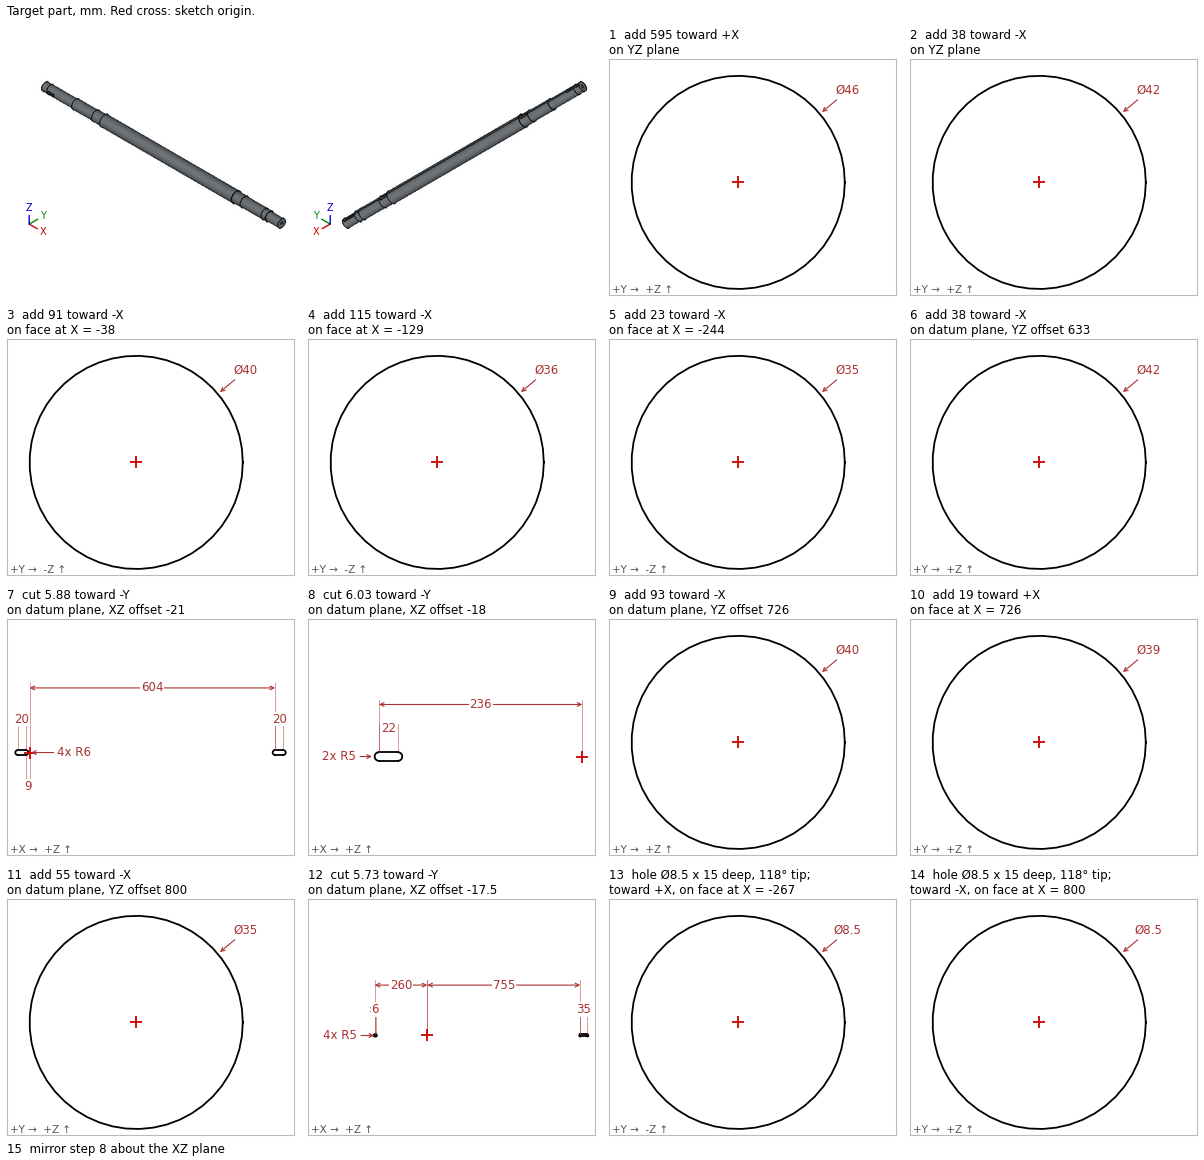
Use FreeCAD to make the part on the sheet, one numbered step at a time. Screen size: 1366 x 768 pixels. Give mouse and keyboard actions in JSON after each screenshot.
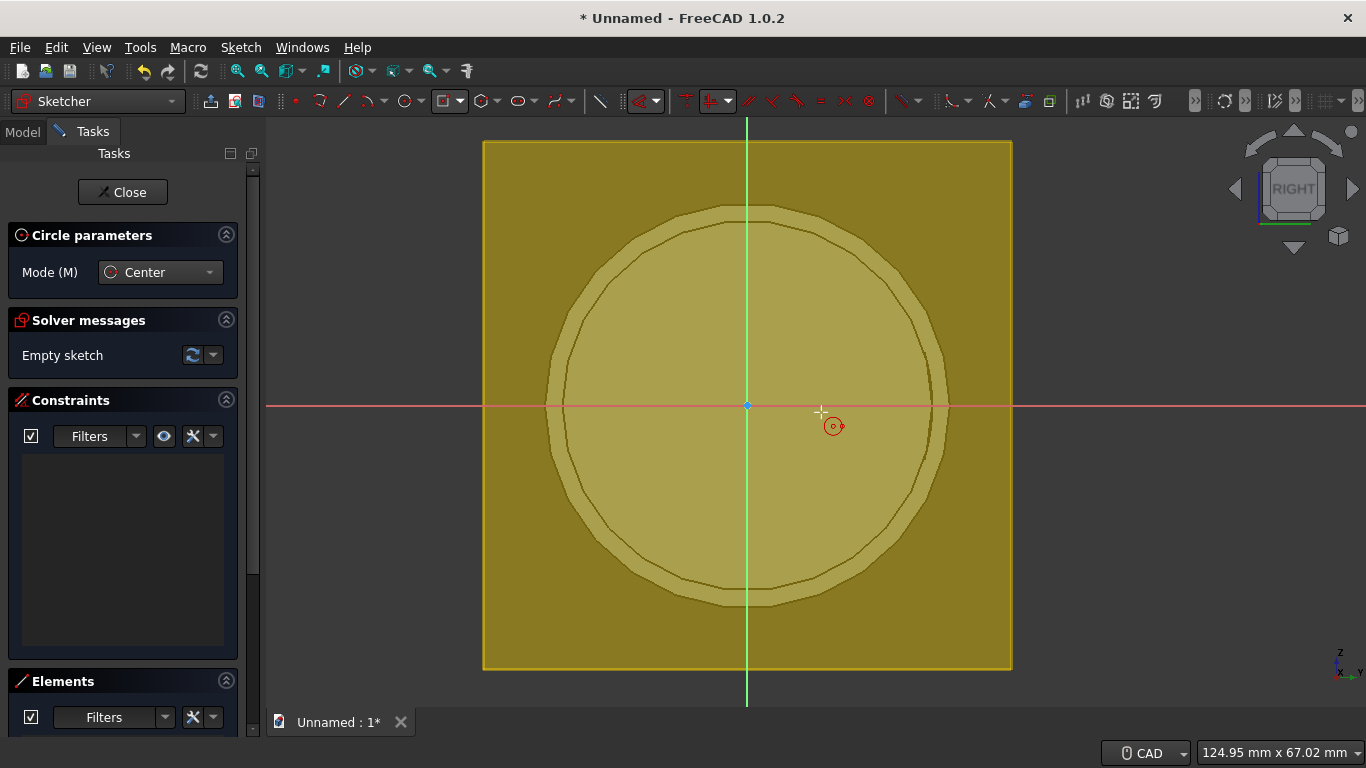
{"action": "left_click", "coordinate": [747, 406]}
{"action": "mouse_move", "coordinate": [872, 281]}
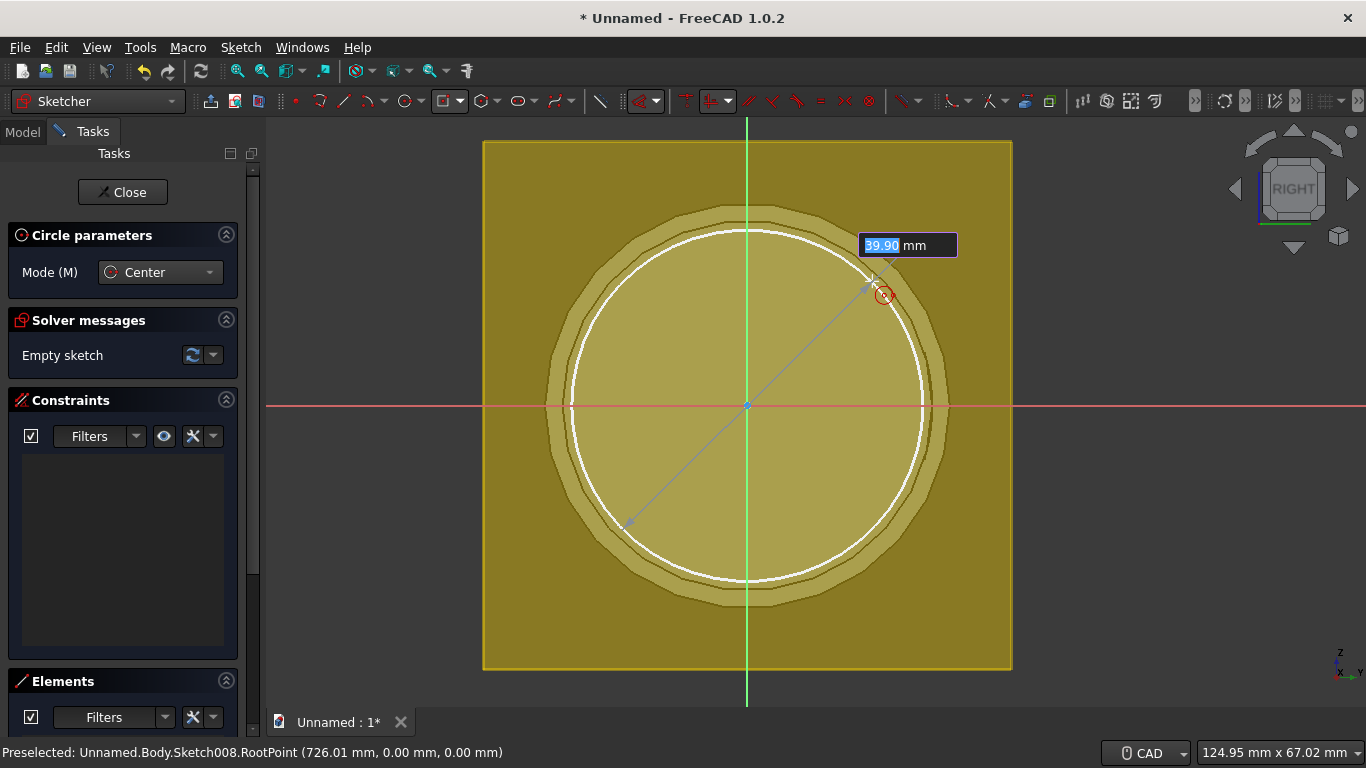
{"action": "type", "text": "40"}
{"action": "key", "text": "Return"}
{"action": "key", "text": "Escape"}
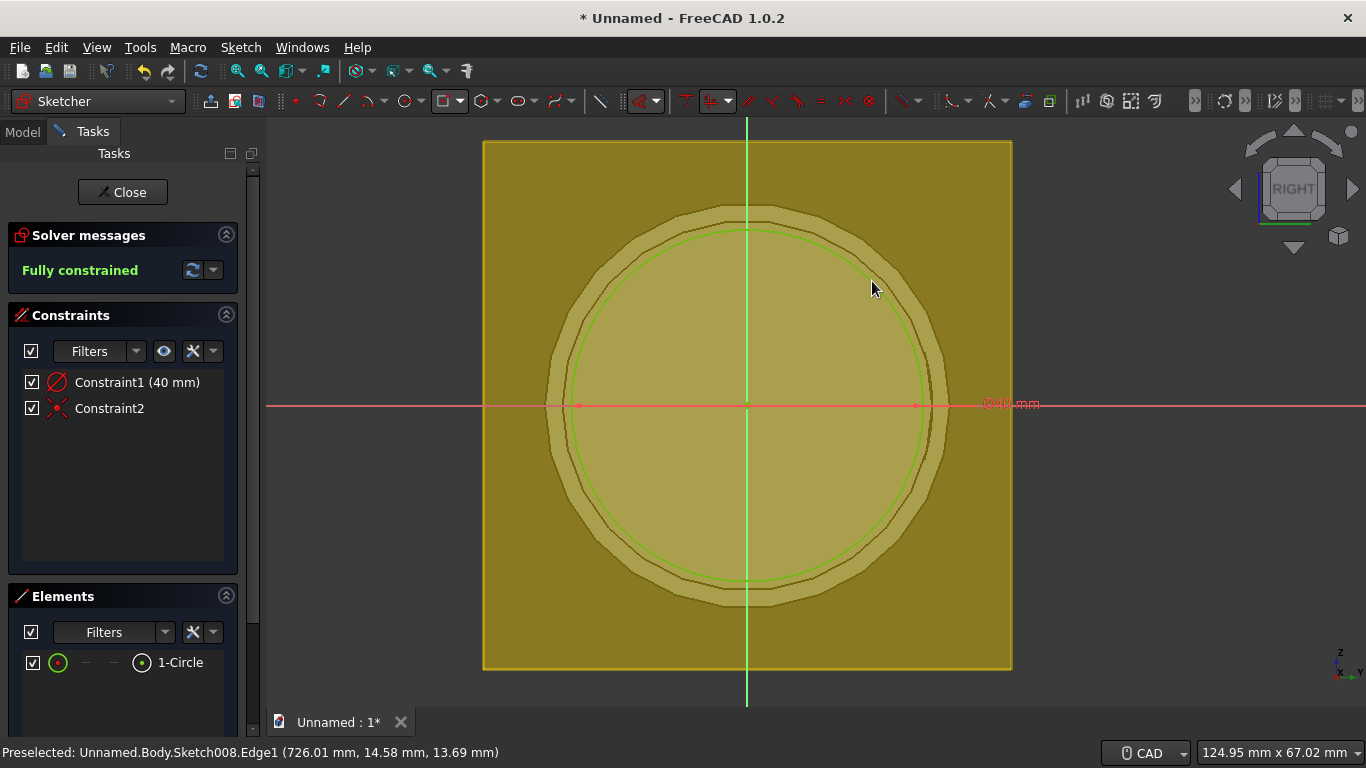
{"action": "left_click", "coordinate": [123, 192]}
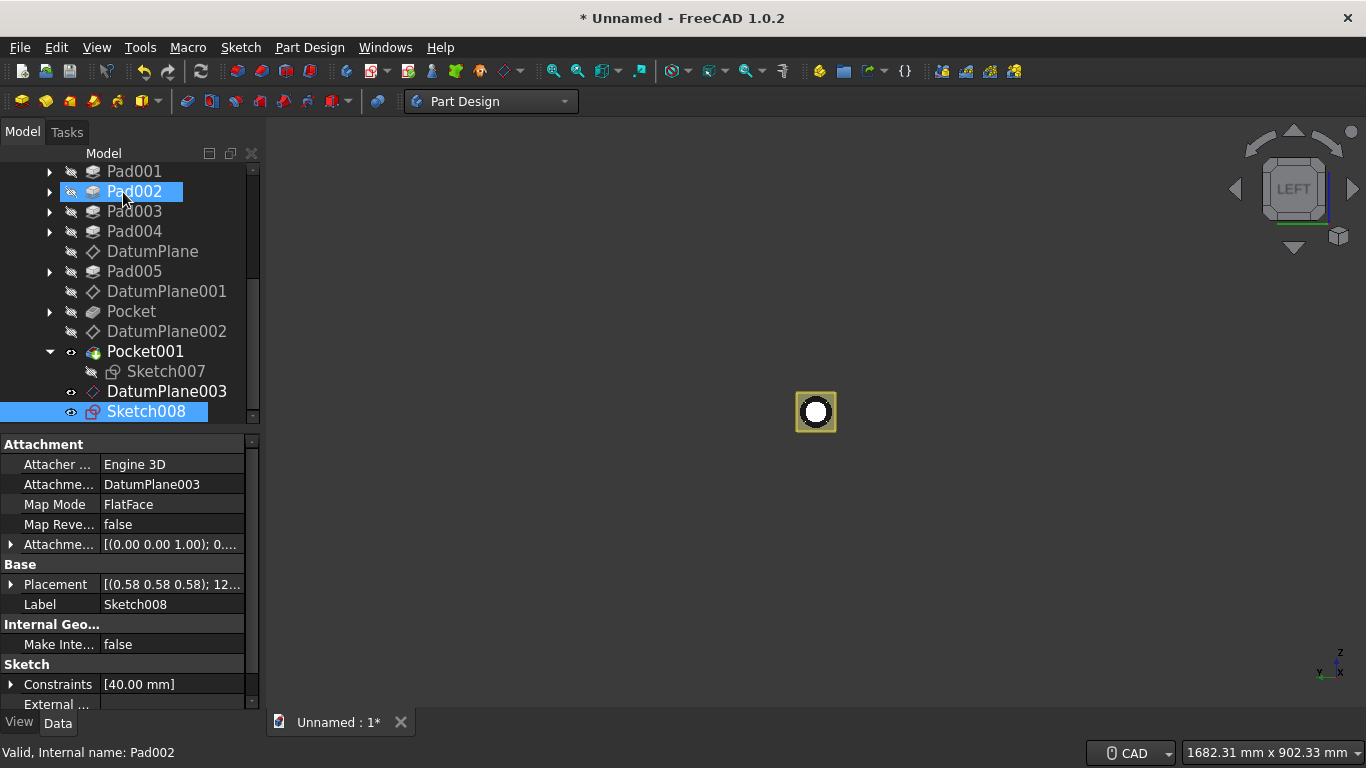
{"action": "left_click", "coordinate": [22, 102]}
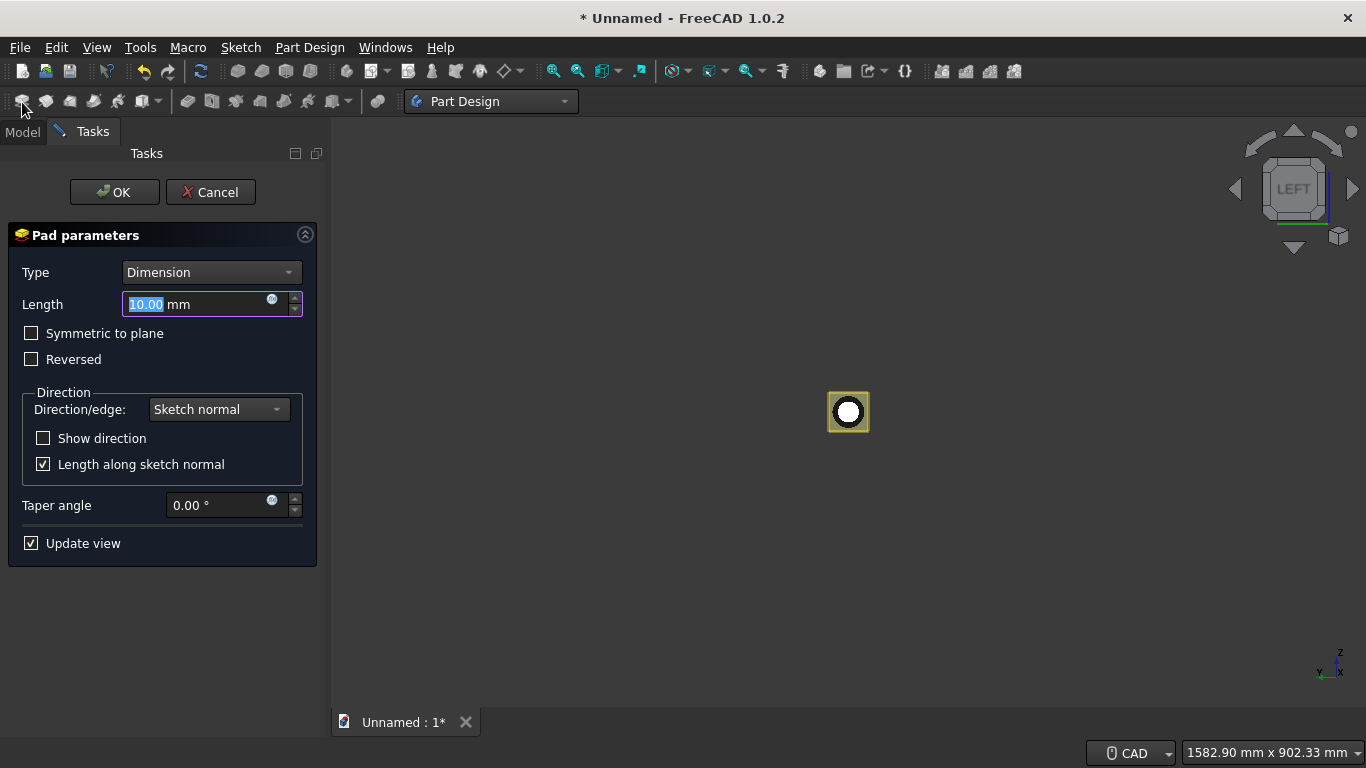
{"action": "type", "text": "93"}
{"action": "key", "text": "Tab"}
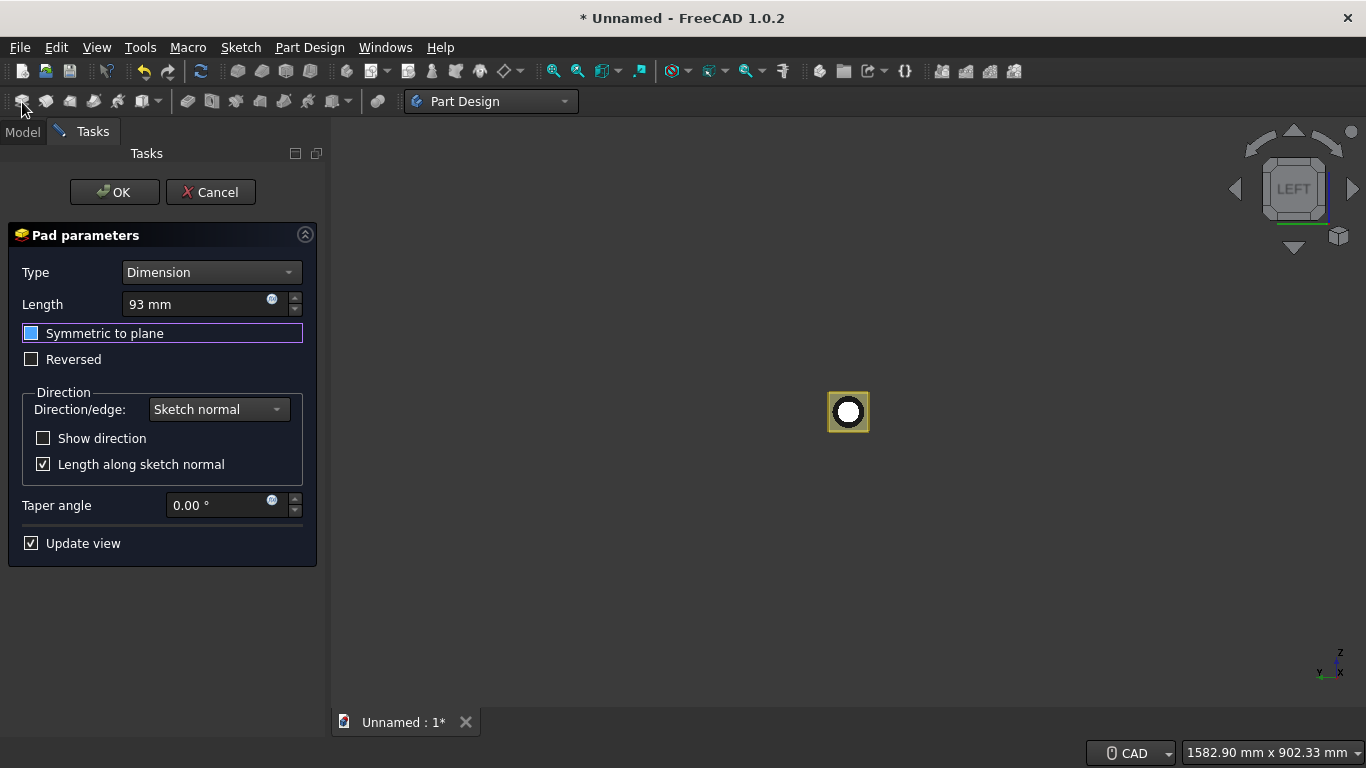
{"action": "left_click", "coordinate": [30, 359]}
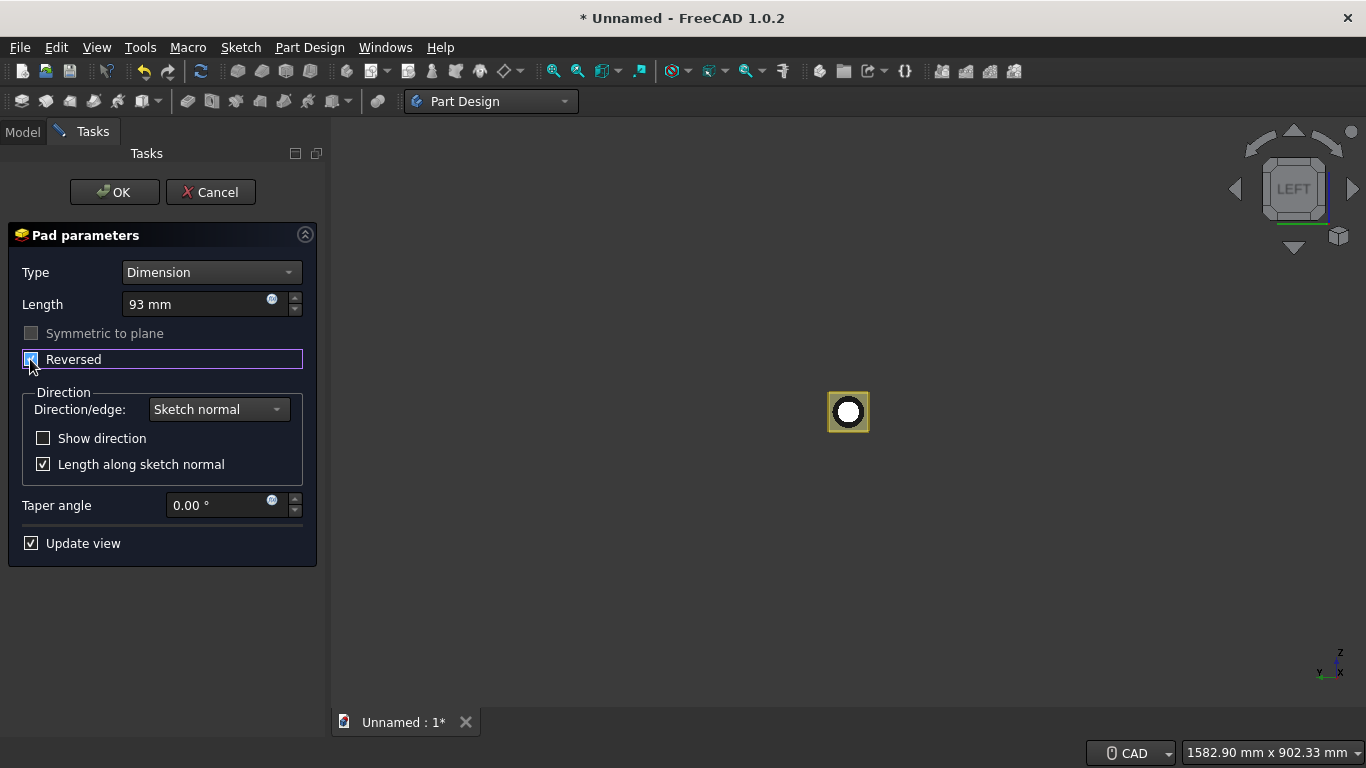
{"action": "left_click", "coordinate": [115, 192]}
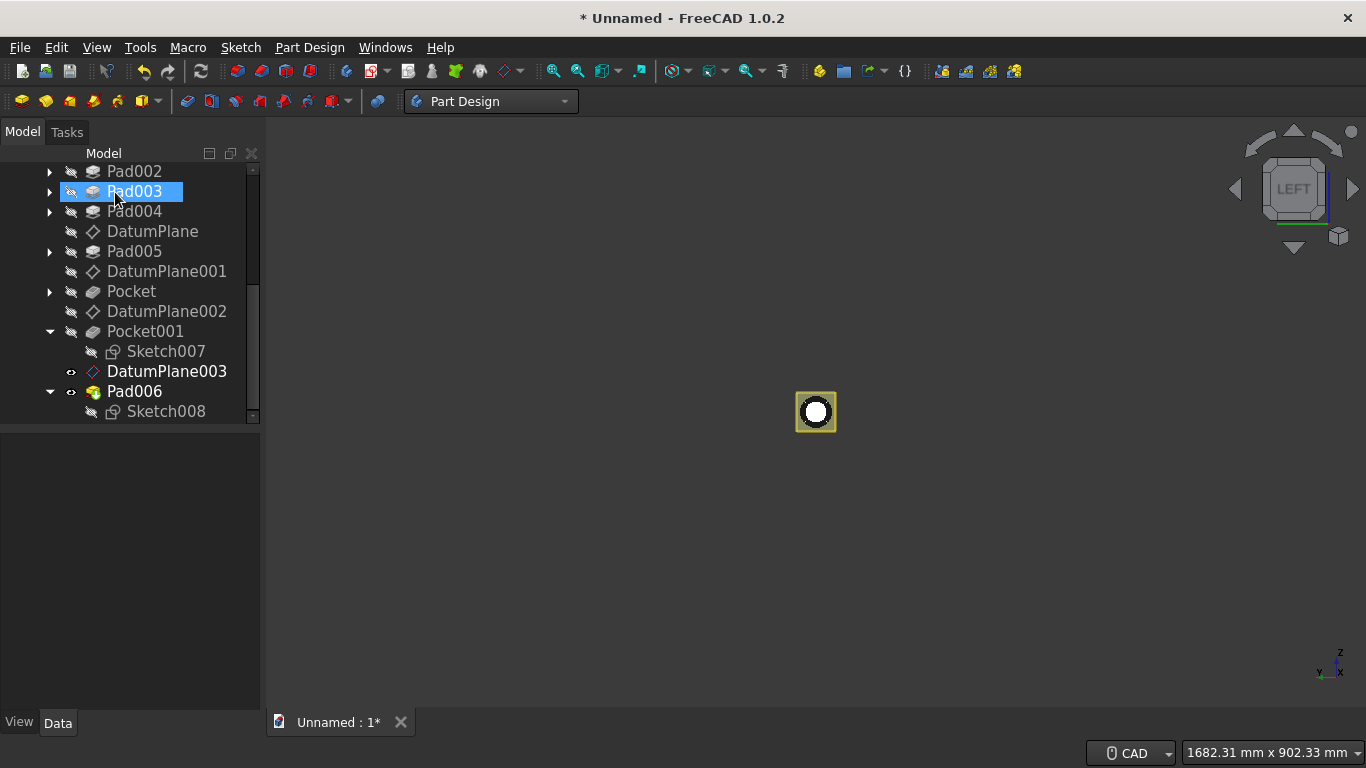
{"action": "left_click", "coordinate": [116, 372]}
{"action": "key", "text": "space"}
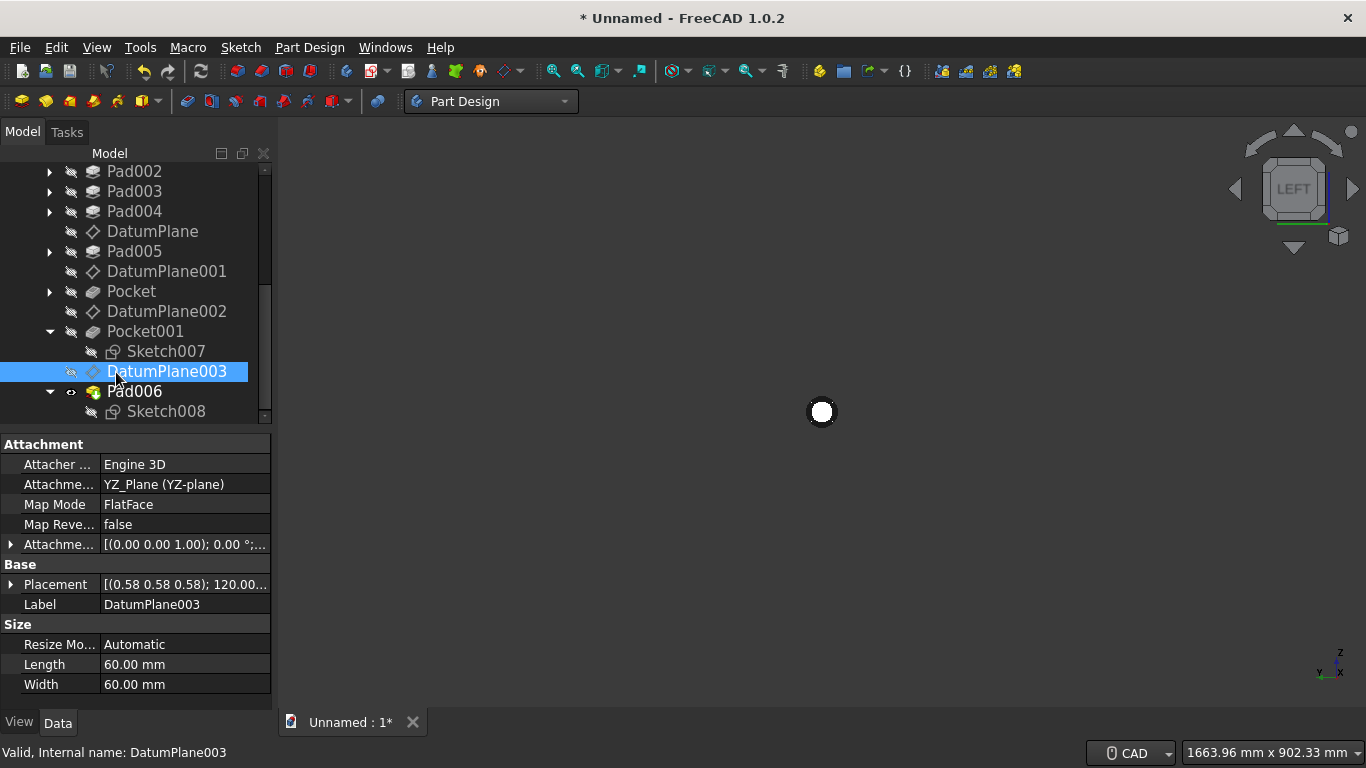
{"action": "key", "text": "v f"}